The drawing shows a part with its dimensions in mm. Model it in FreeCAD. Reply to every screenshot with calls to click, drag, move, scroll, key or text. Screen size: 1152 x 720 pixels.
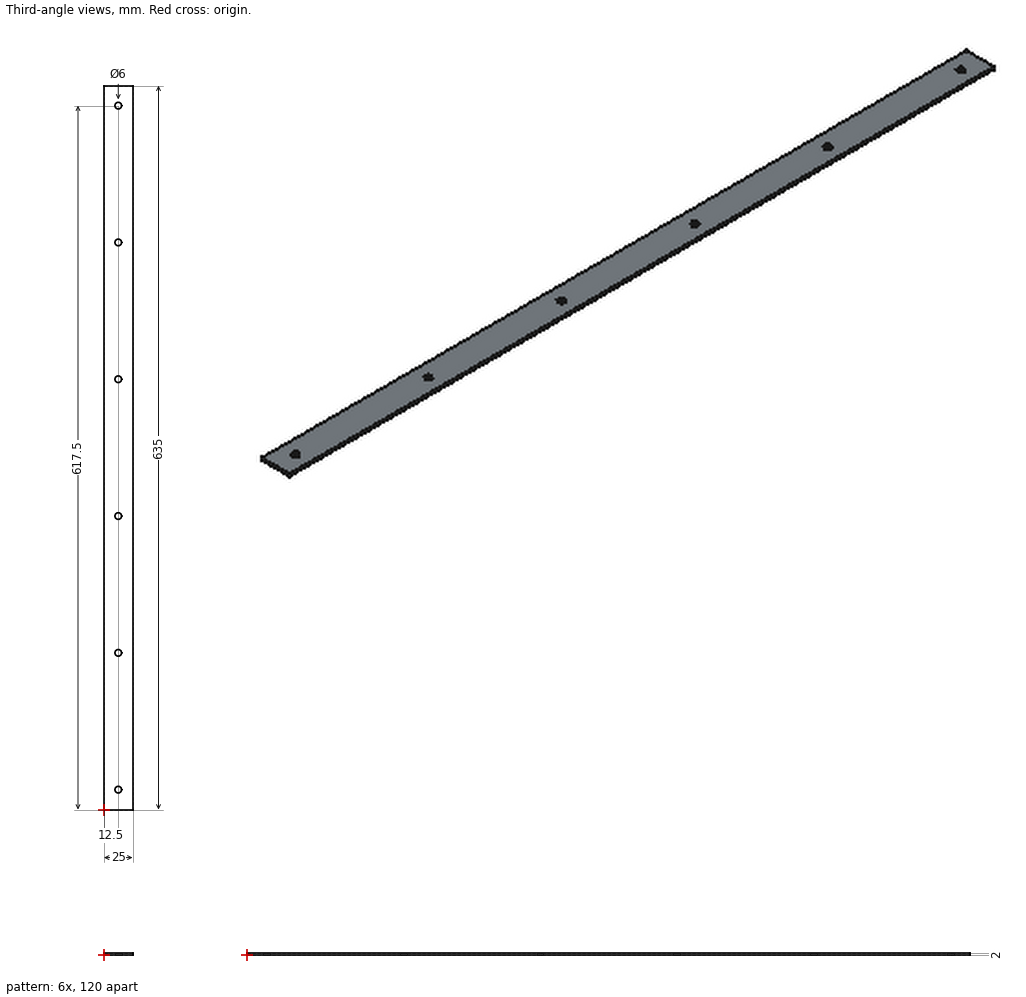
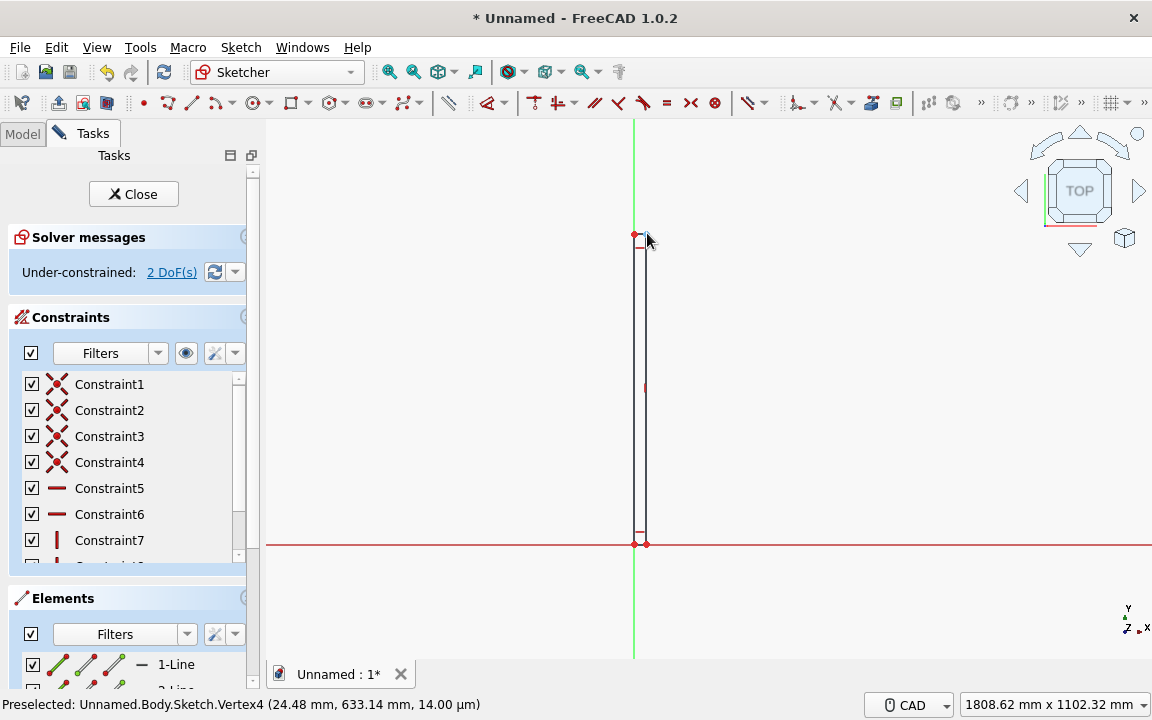
scroll(640, 545, up, 6)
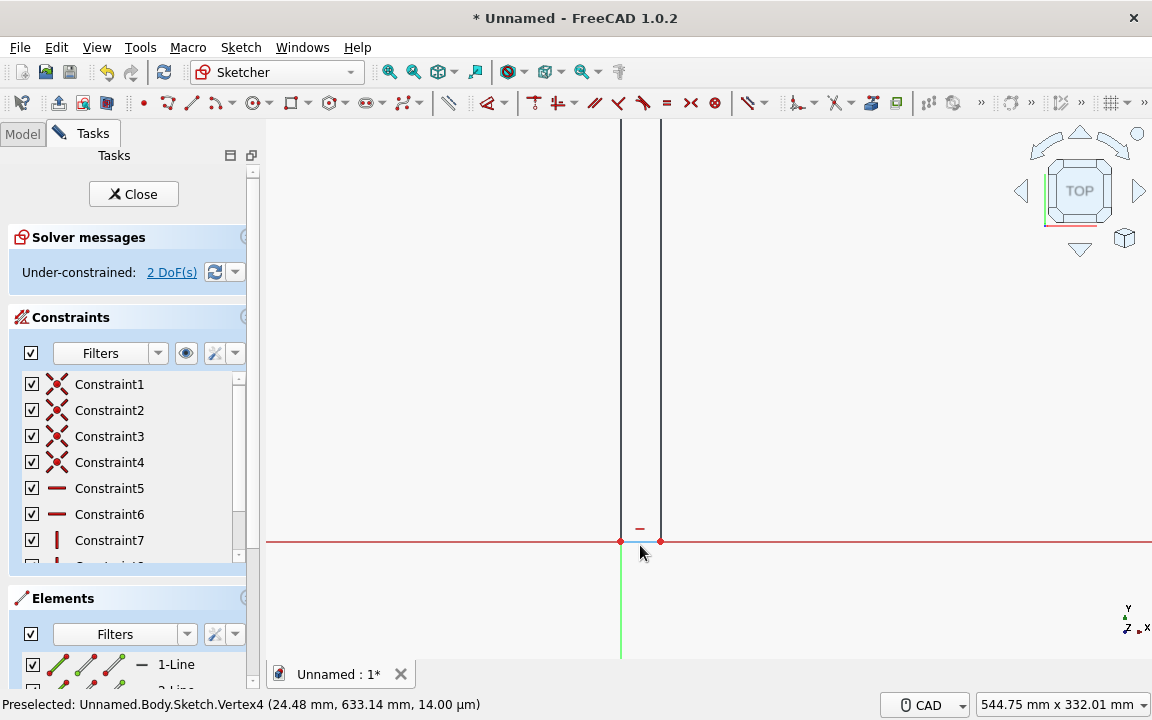
click(641, 542)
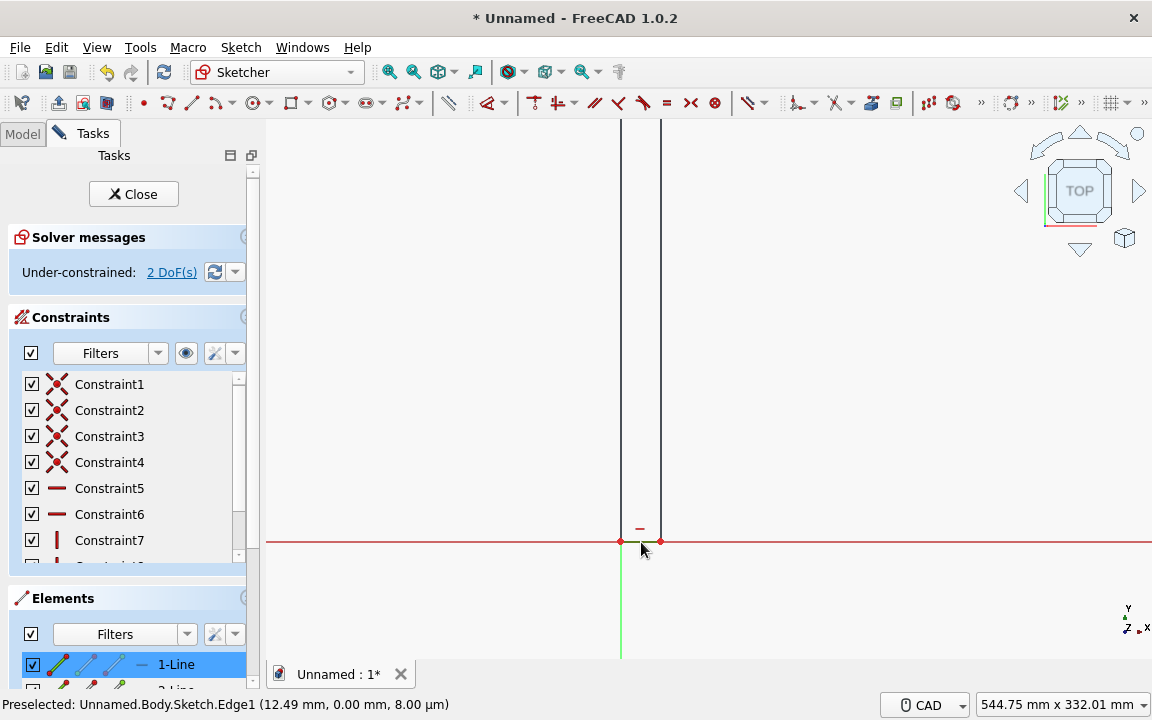
click(506, 104)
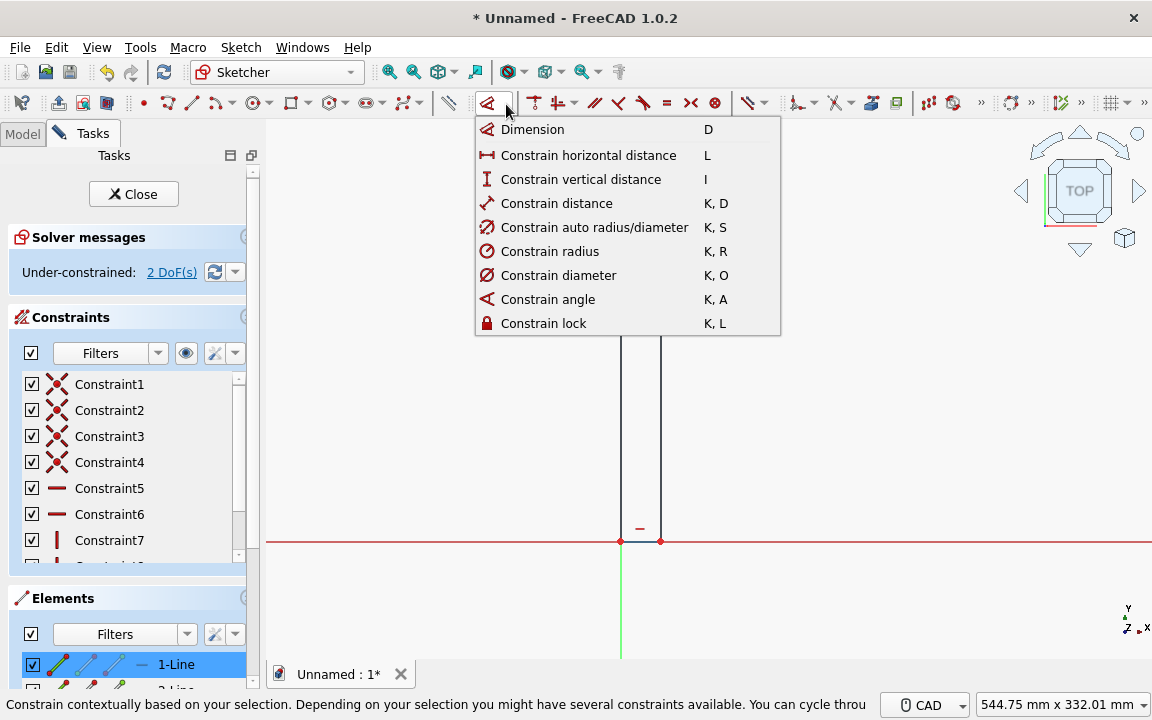
click(628, 155)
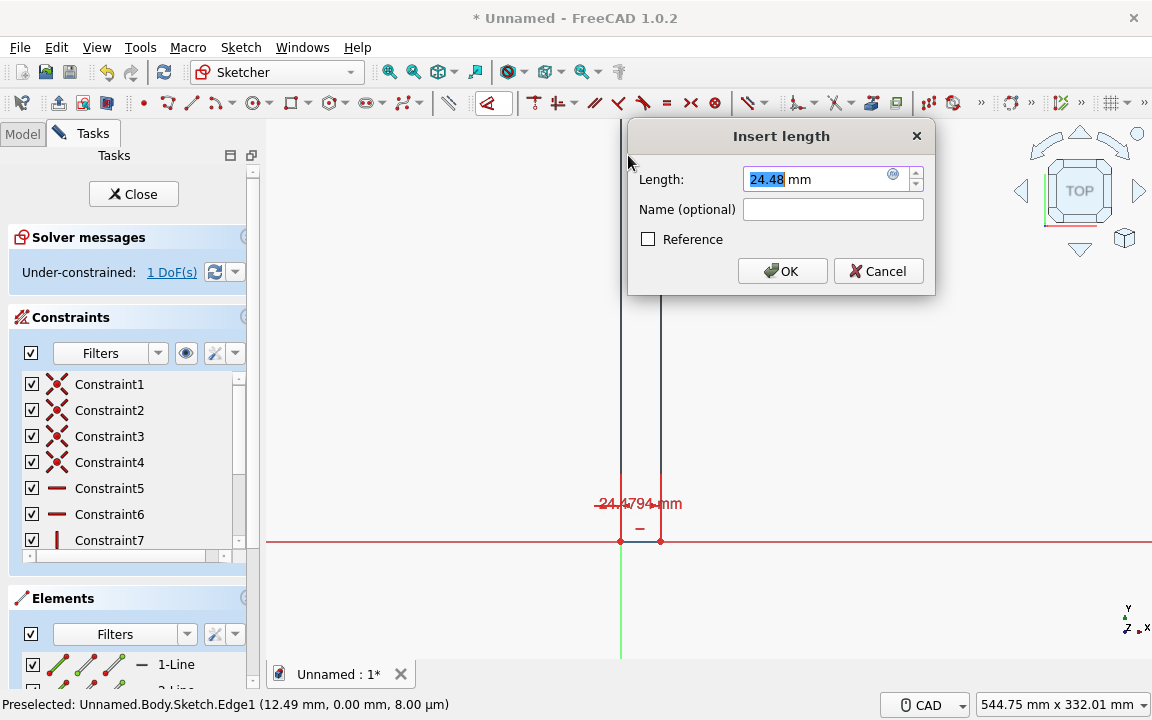
text(25)
key(Return)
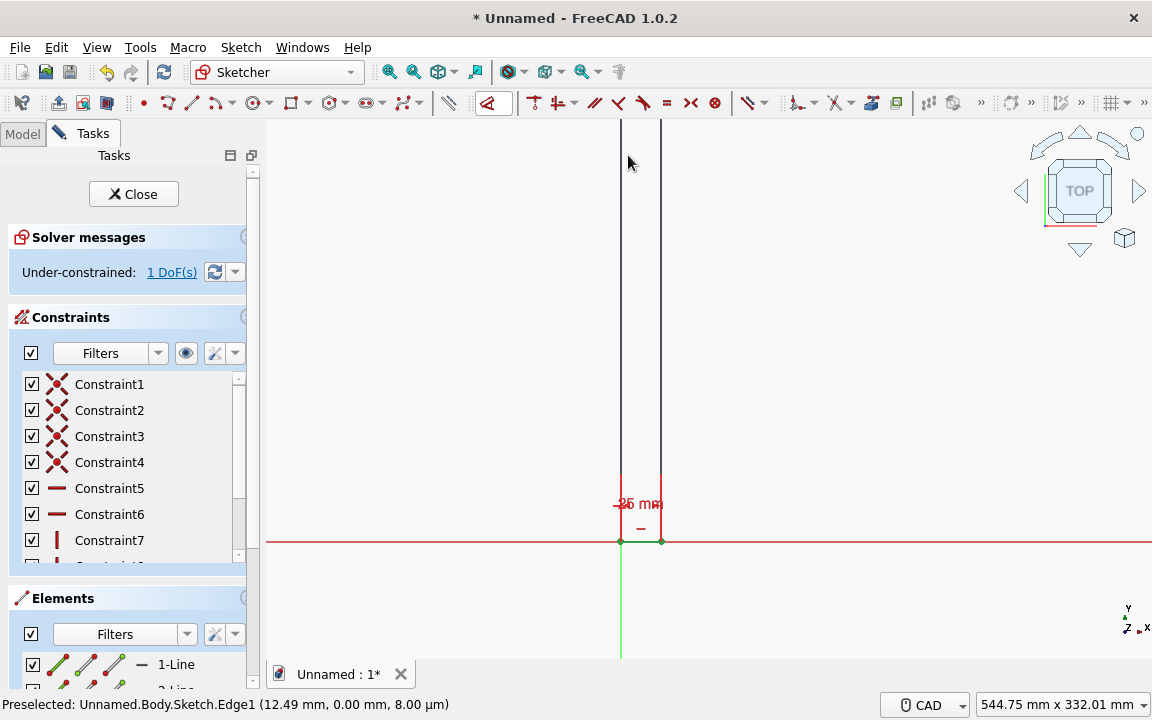
click(661, 233)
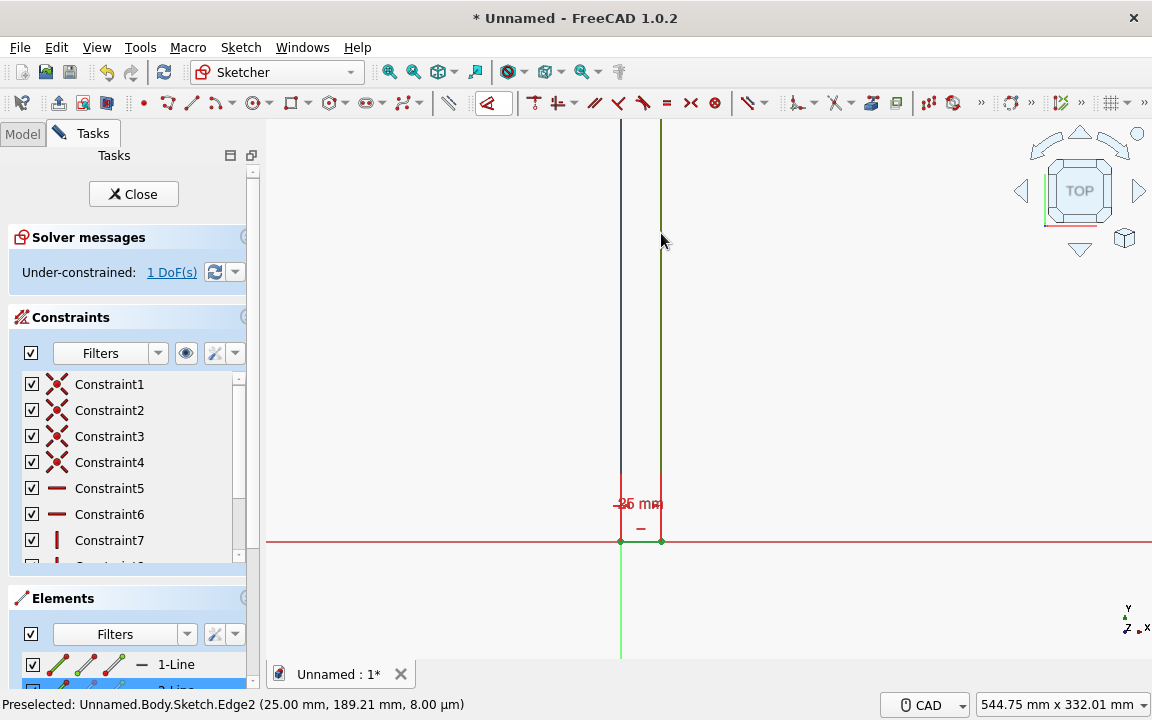
click(506, 104)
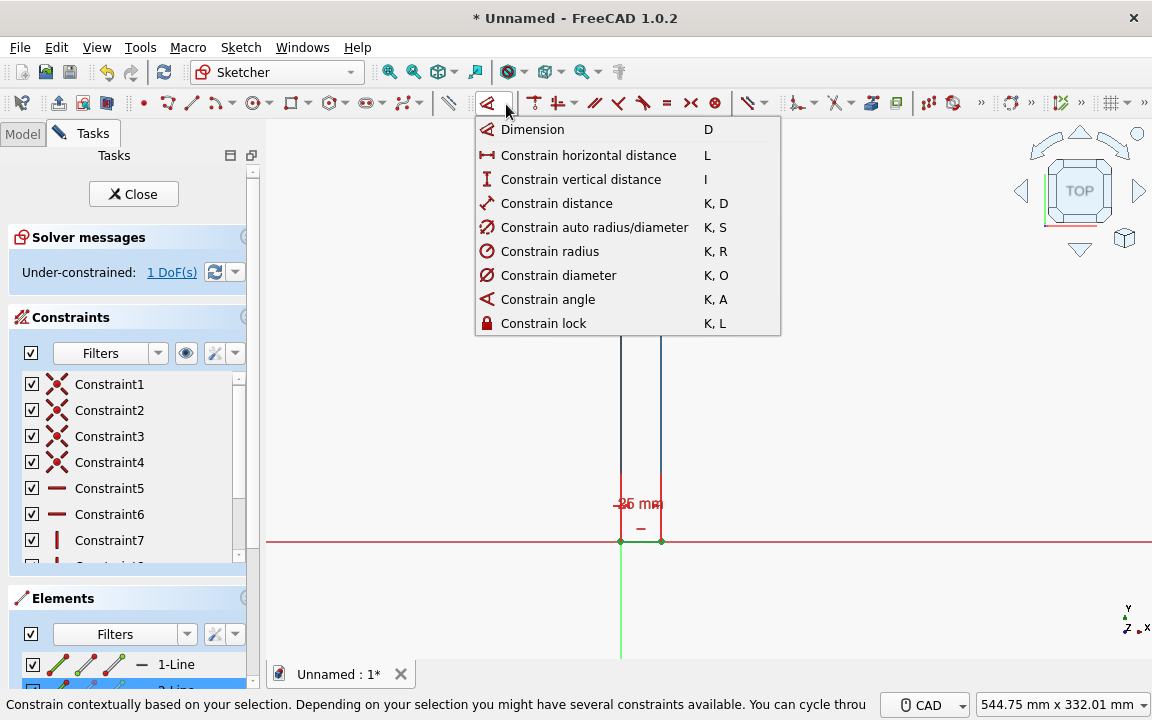
click(628, 179)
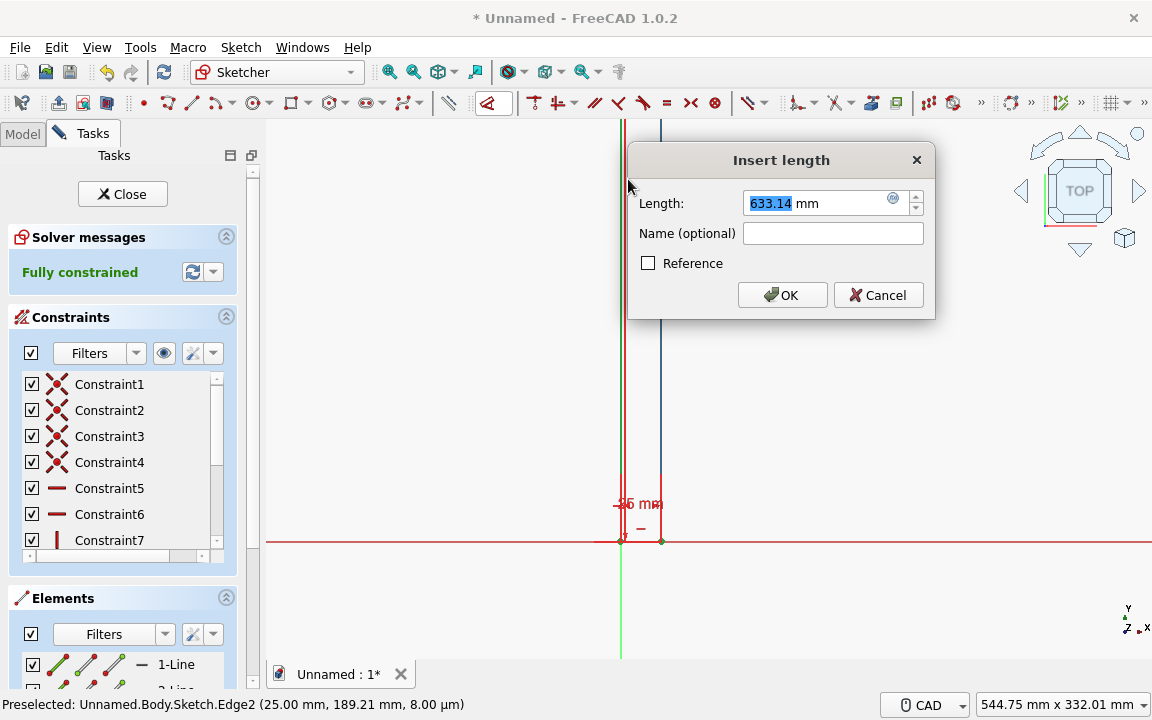
text(635)
key(Return)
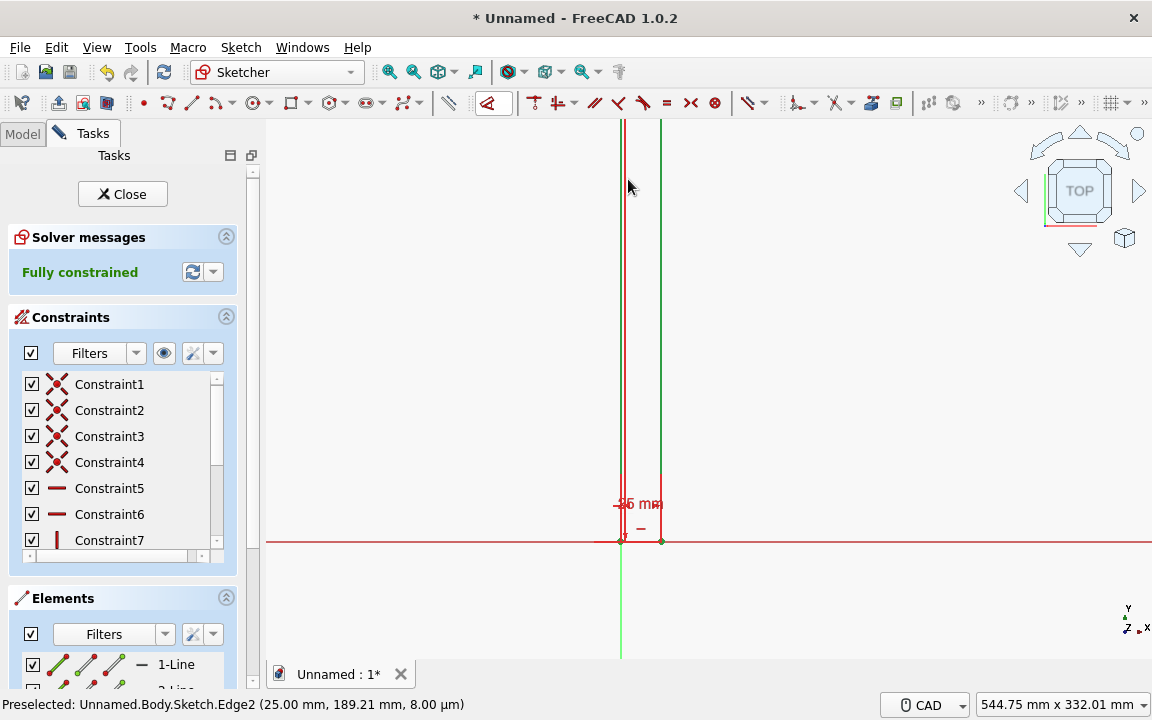
click(123, 194)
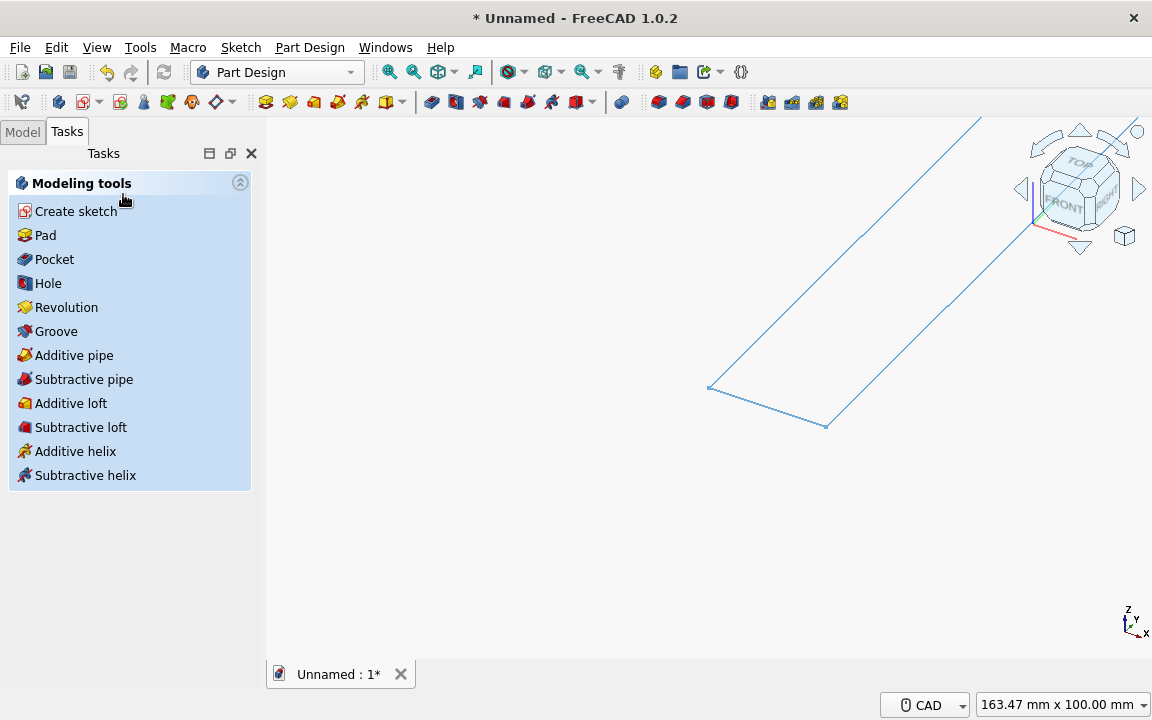
click(266, 102)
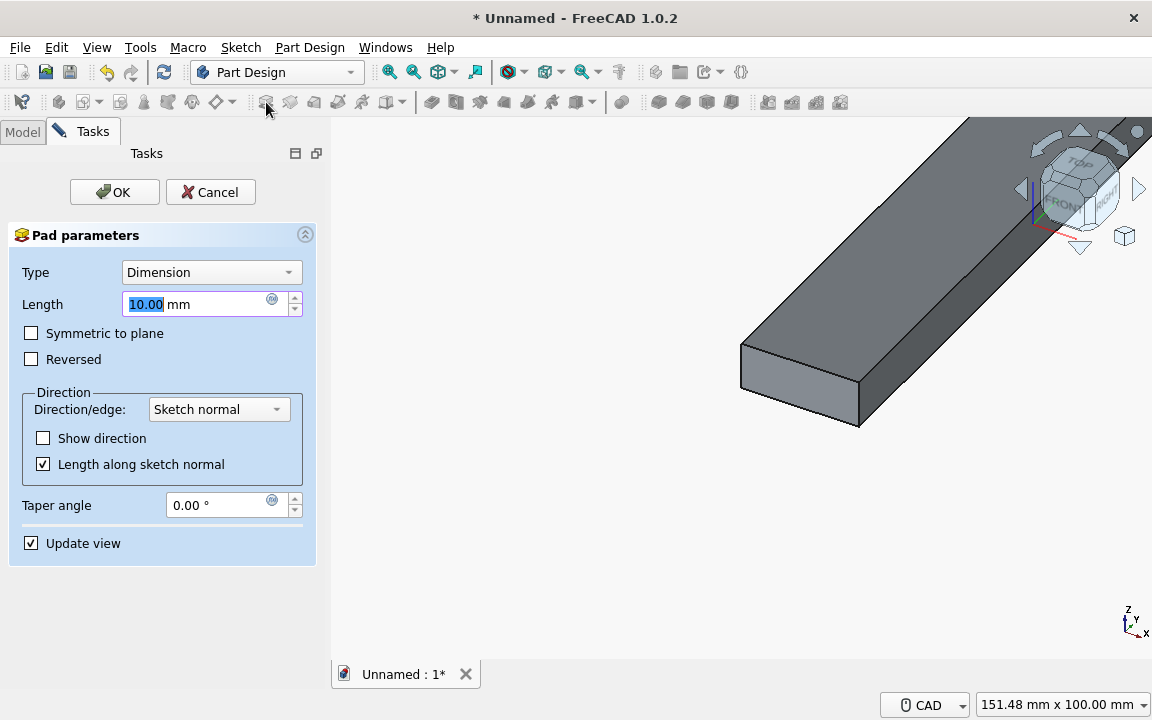
text(2)
key(Tab)